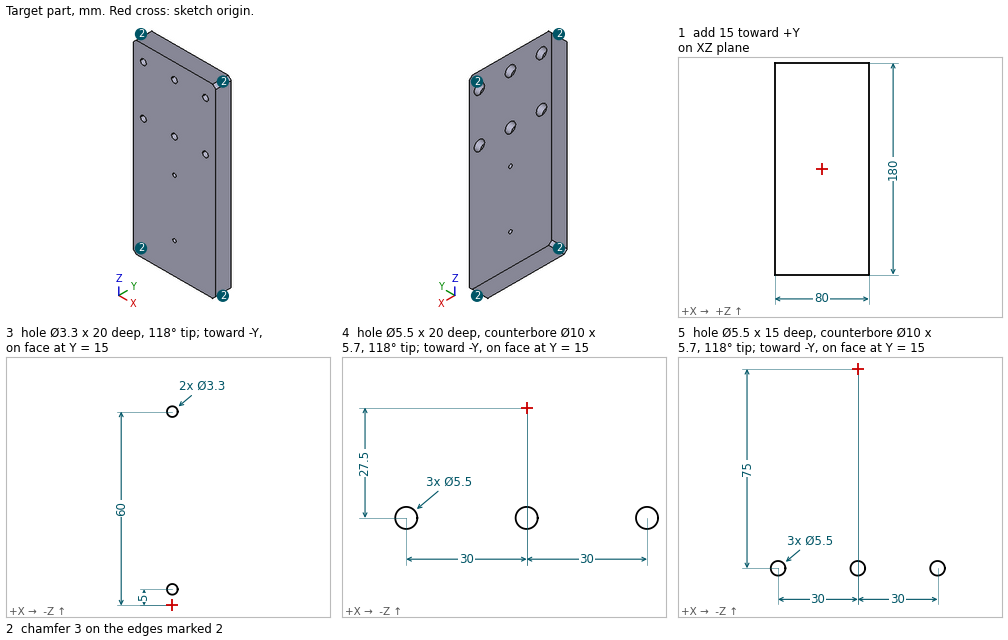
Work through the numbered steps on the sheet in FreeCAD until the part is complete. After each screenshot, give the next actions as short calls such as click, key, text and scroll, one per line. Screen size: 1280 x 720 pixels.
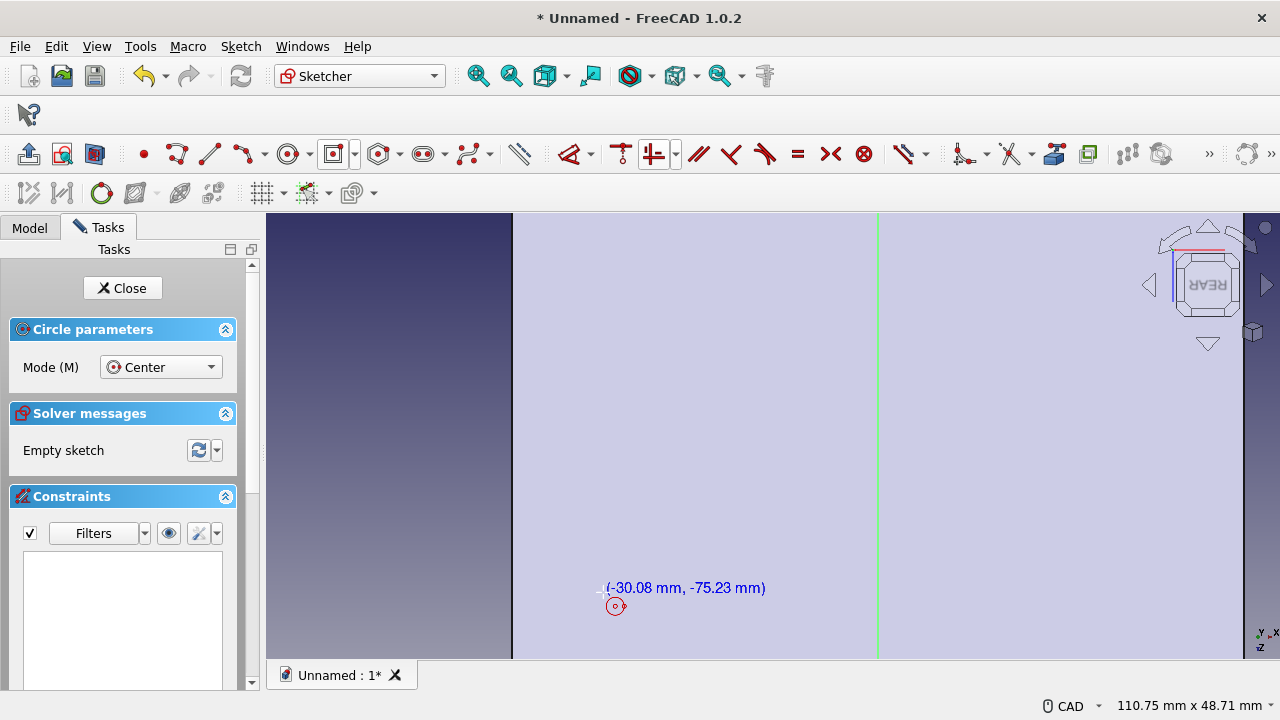
click(603, 591)
click(621, 573)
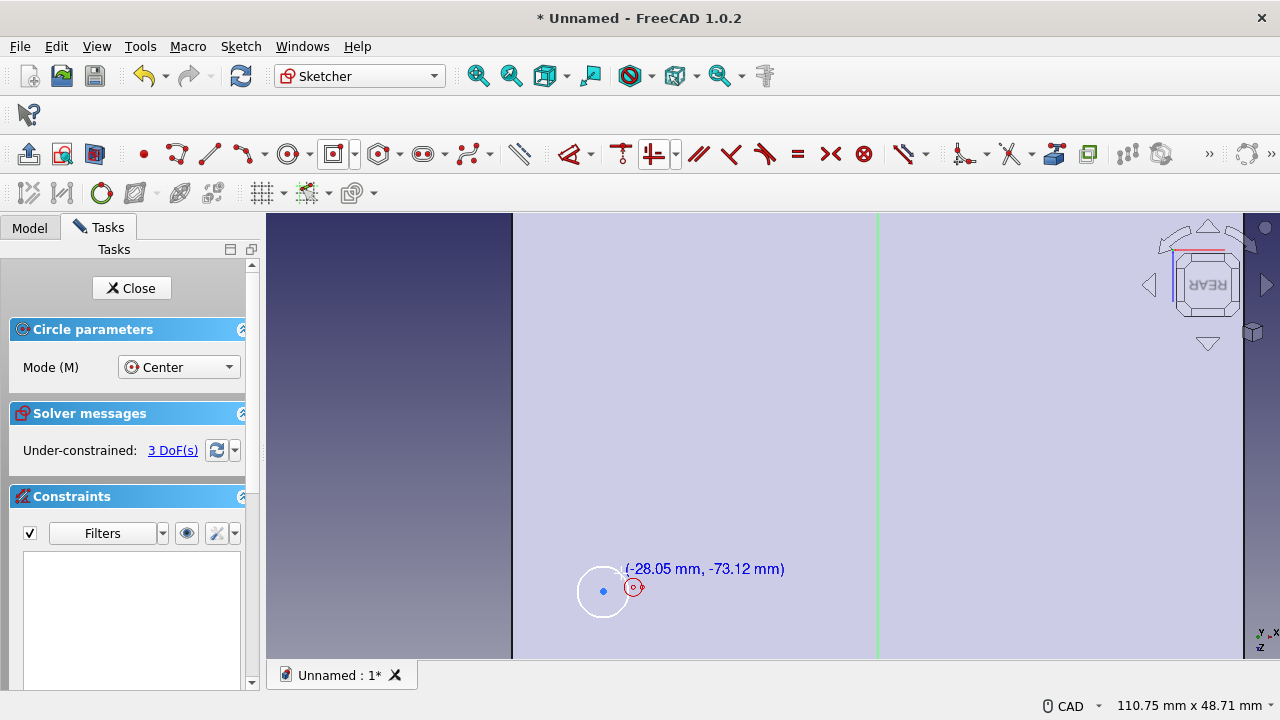
click(878, 591)
click(896, 573)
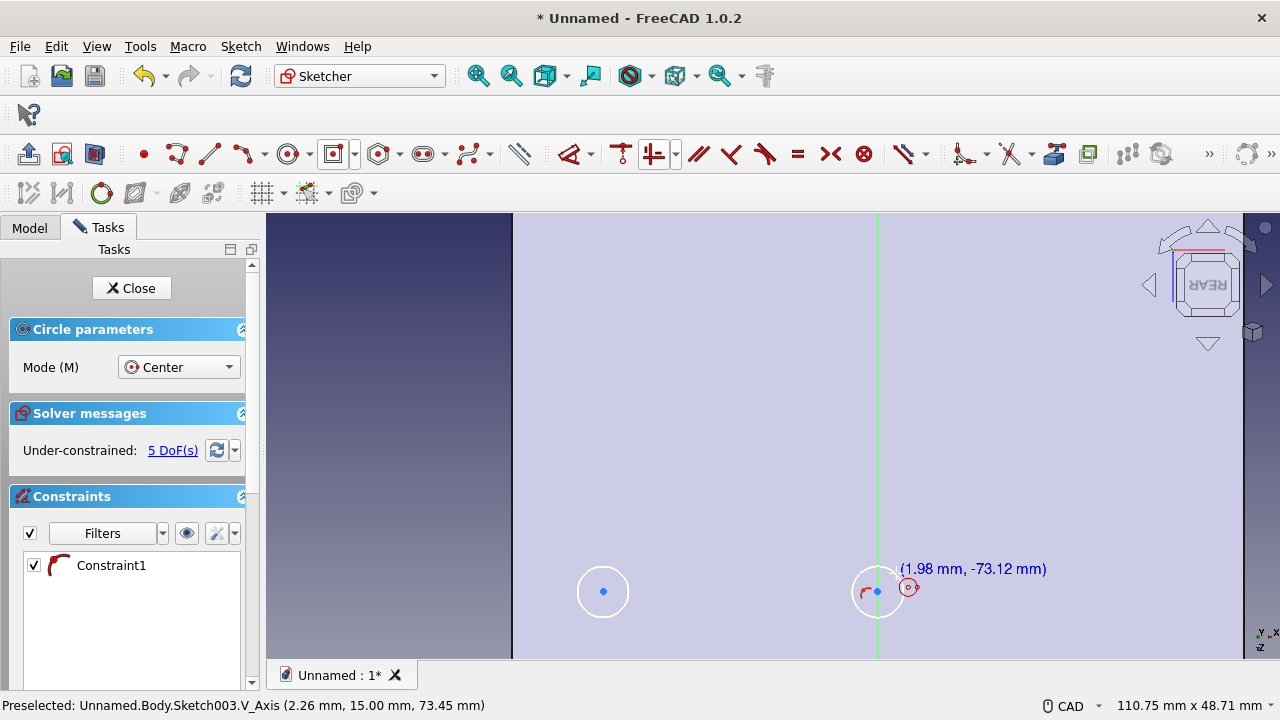
scroll(604, 538, down, 5)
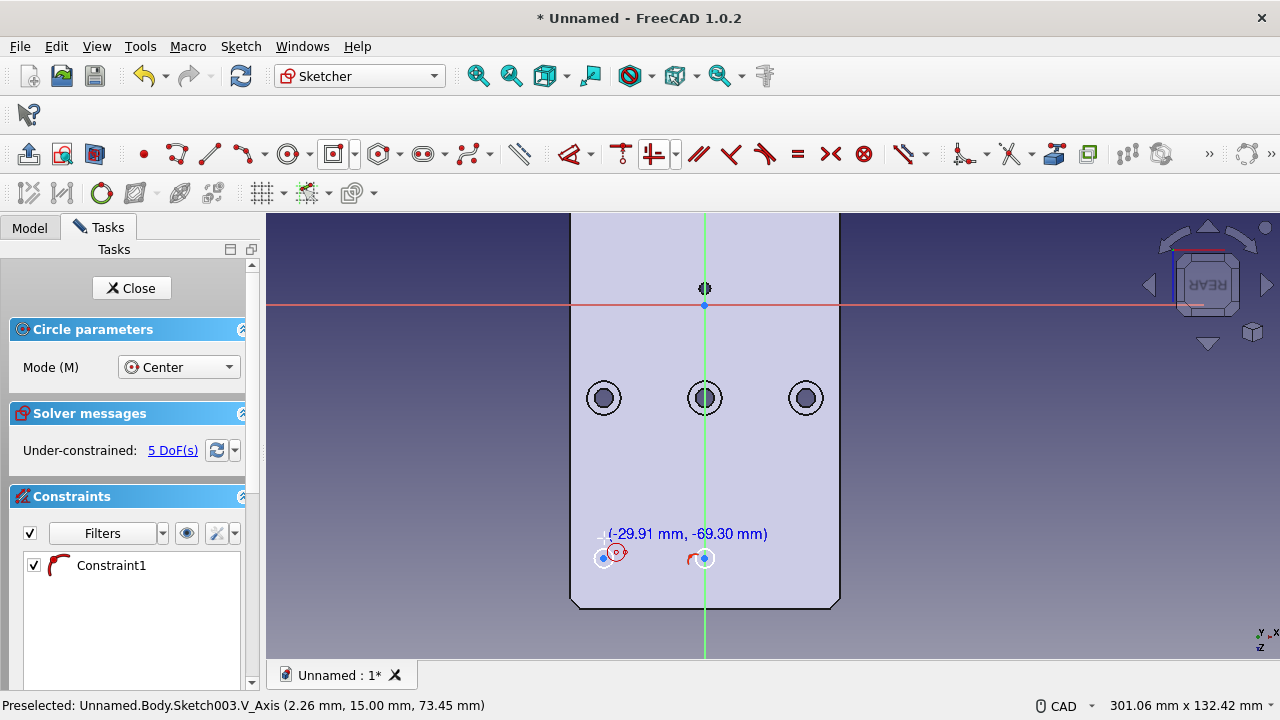
scroll(806, 558, up, 5)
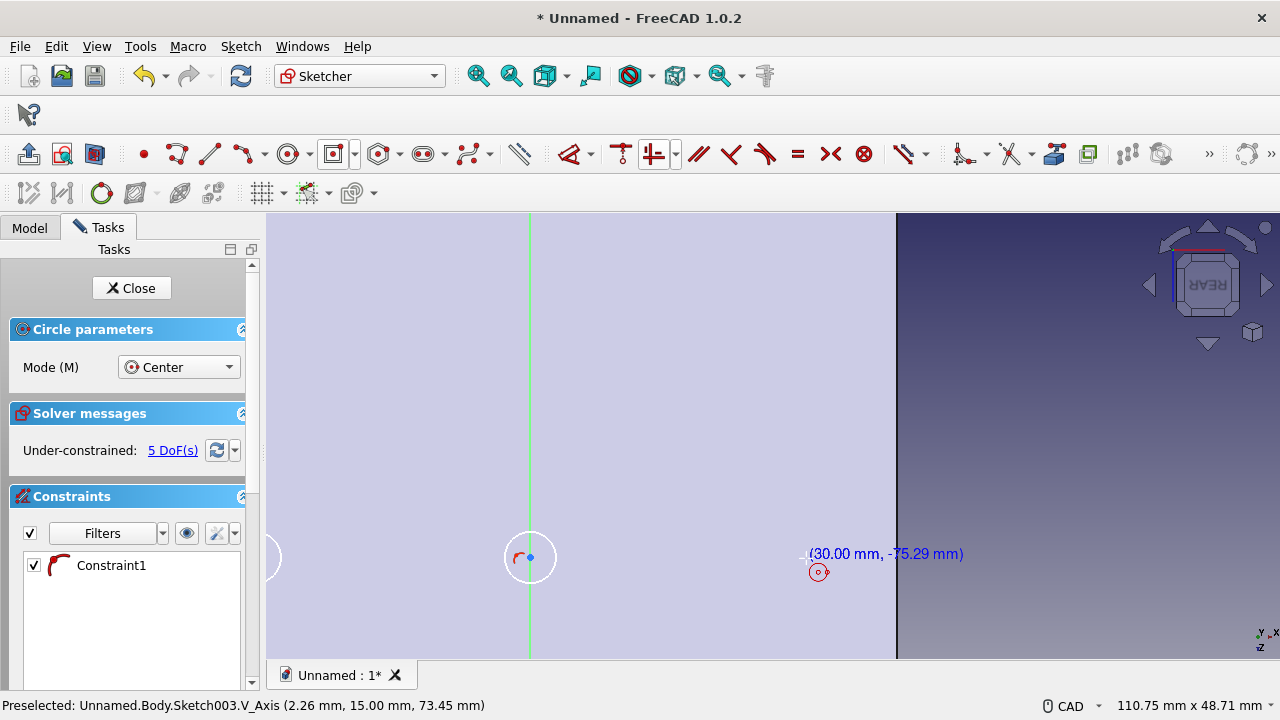
click(805, 557)
click(823, 539)
key(Escape)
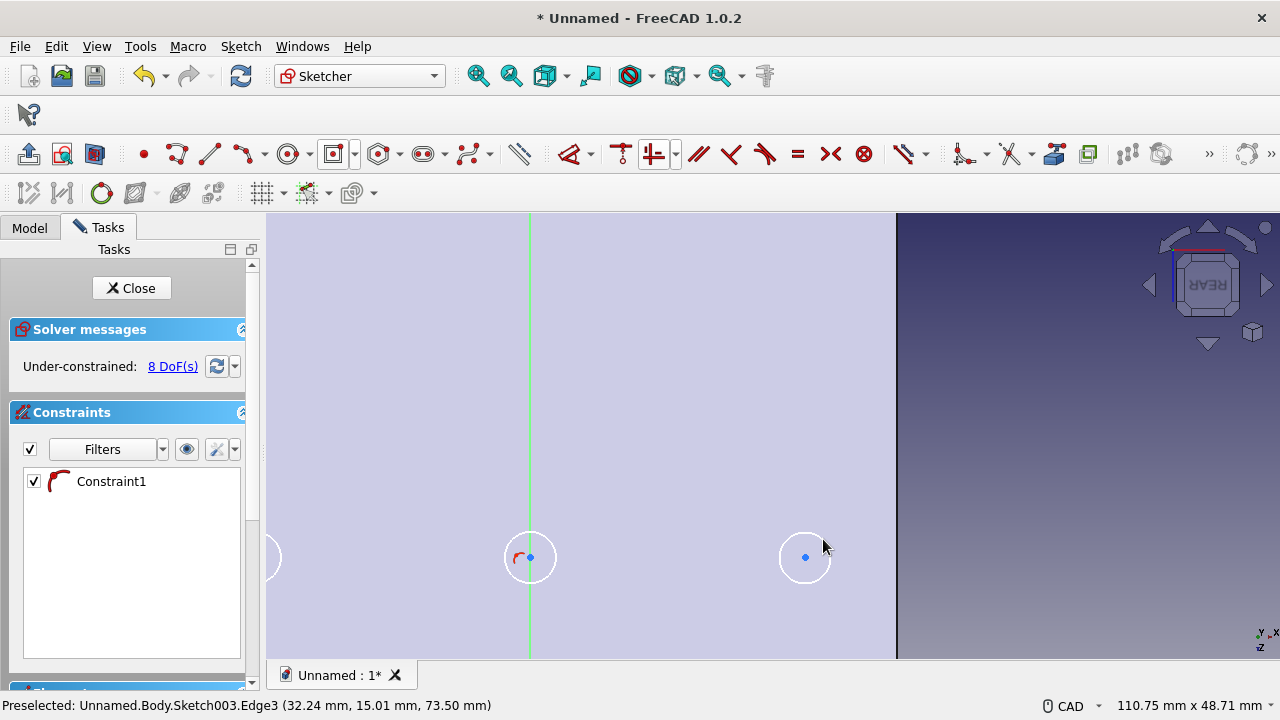
scroll(806, 558, down, 5)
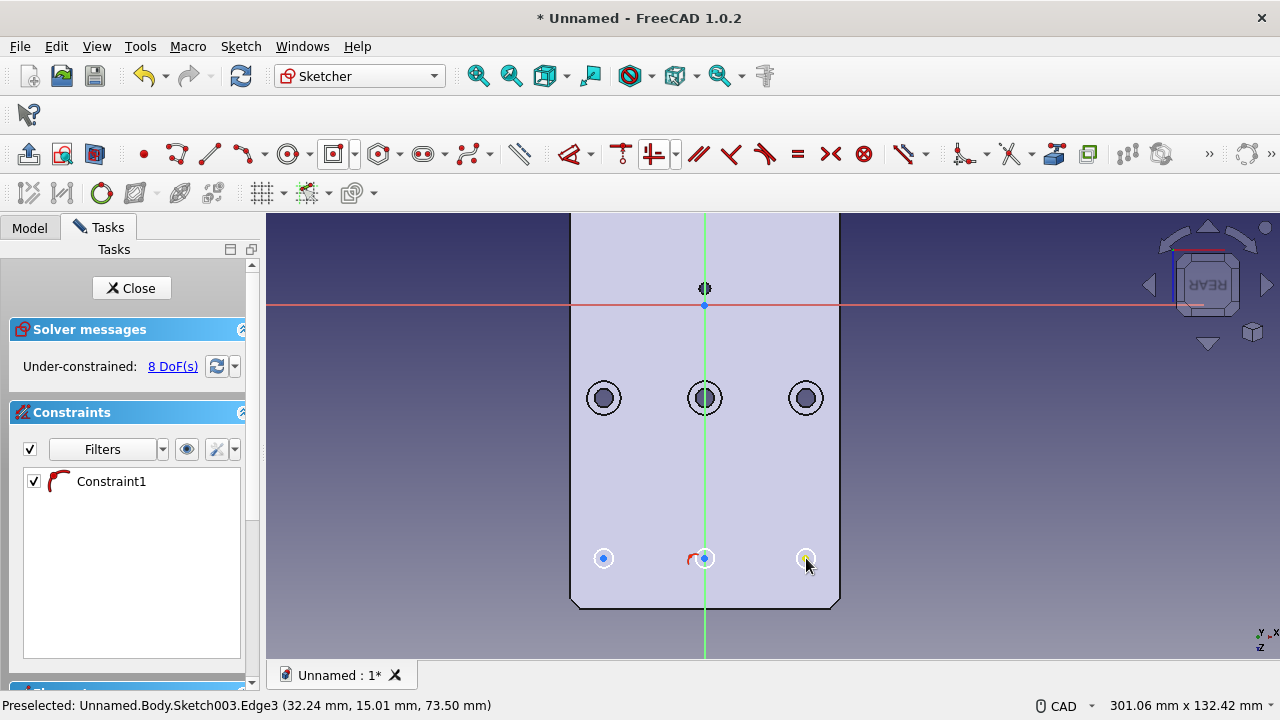
scroll(610, 552, up, 2)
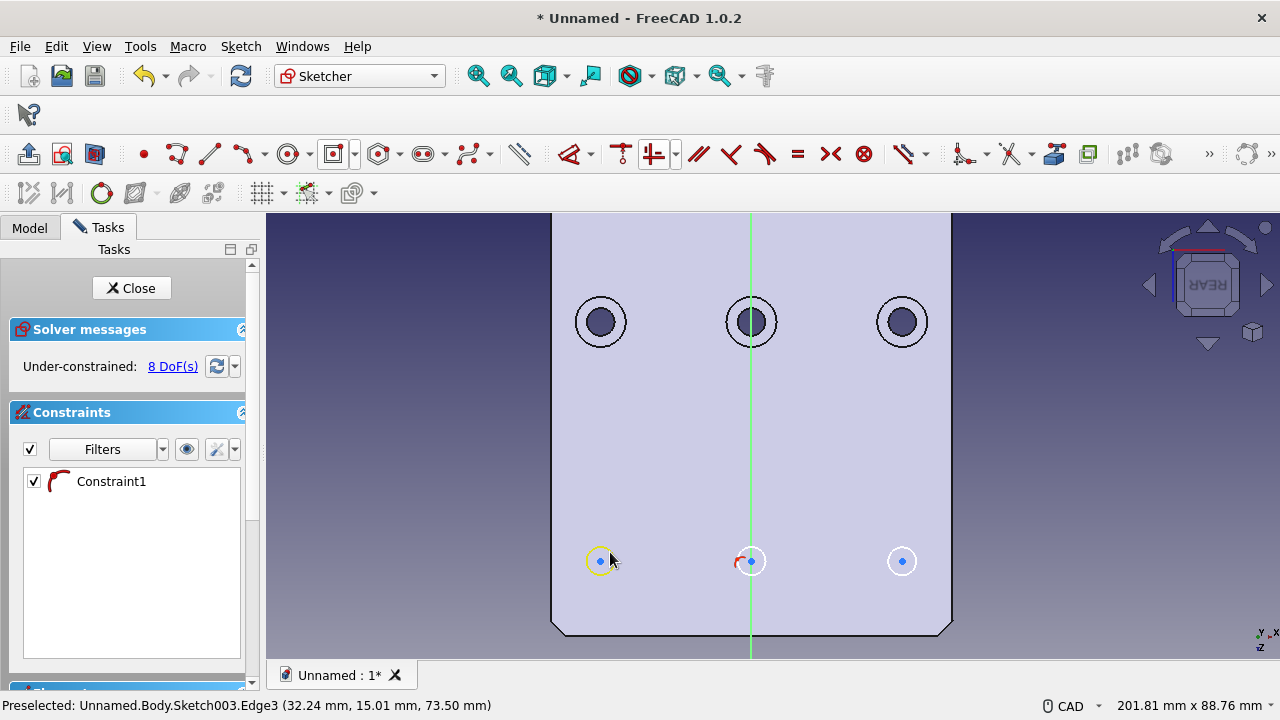
click(610, 551)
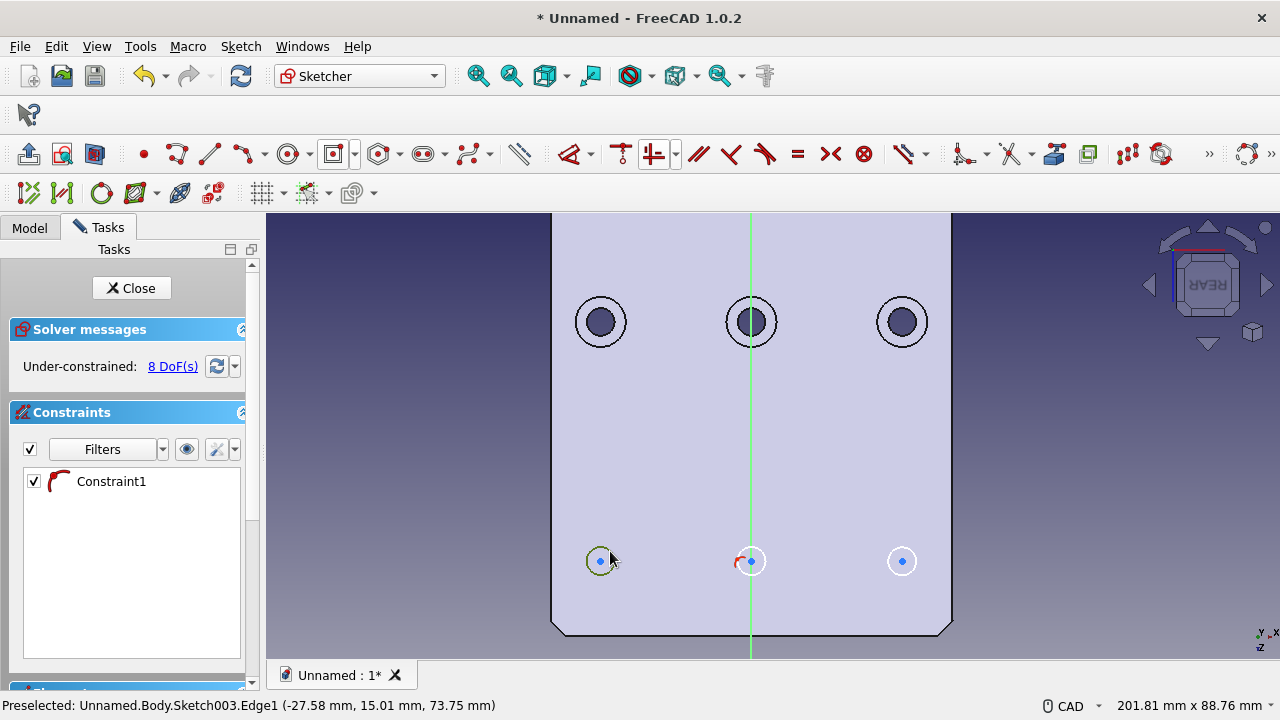
scroll(761, 551, up, 2)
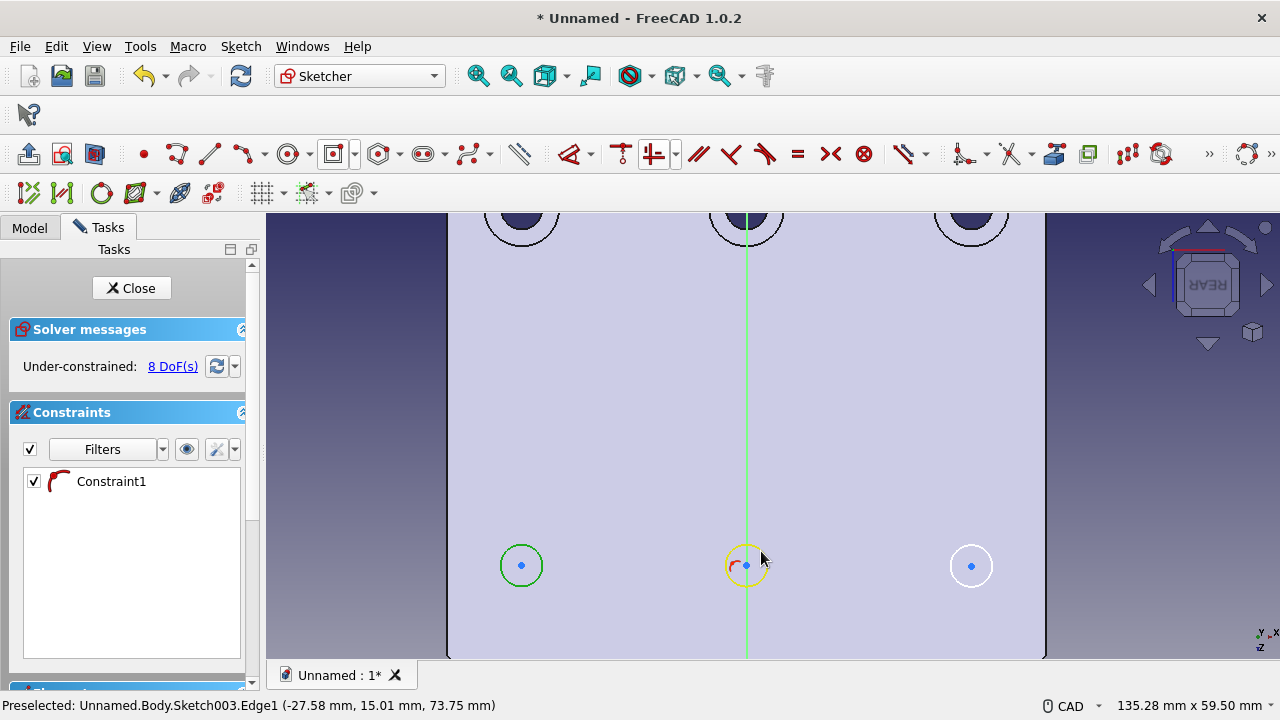
click(761, 551)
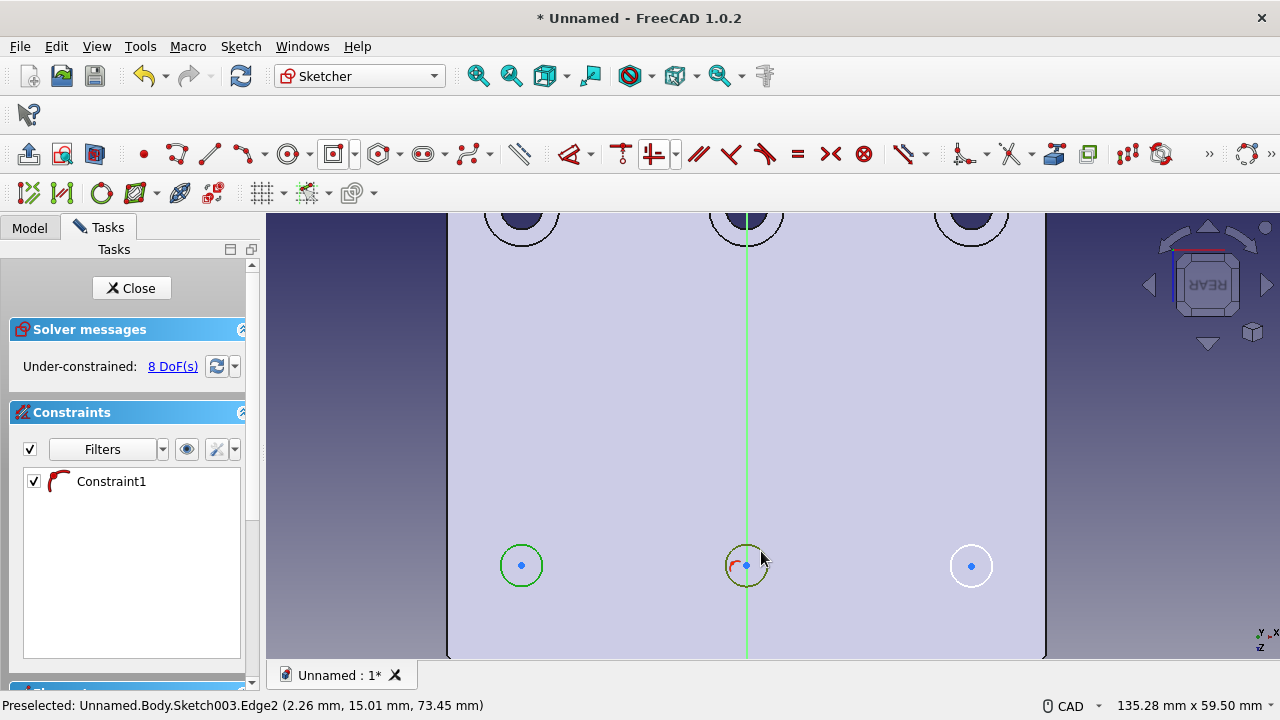
click(986, 551)